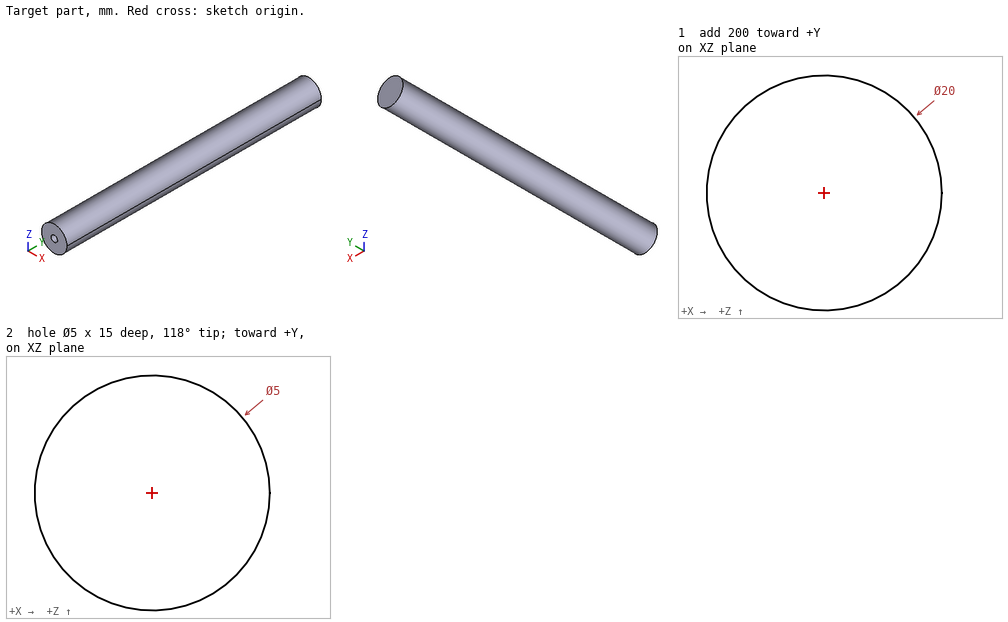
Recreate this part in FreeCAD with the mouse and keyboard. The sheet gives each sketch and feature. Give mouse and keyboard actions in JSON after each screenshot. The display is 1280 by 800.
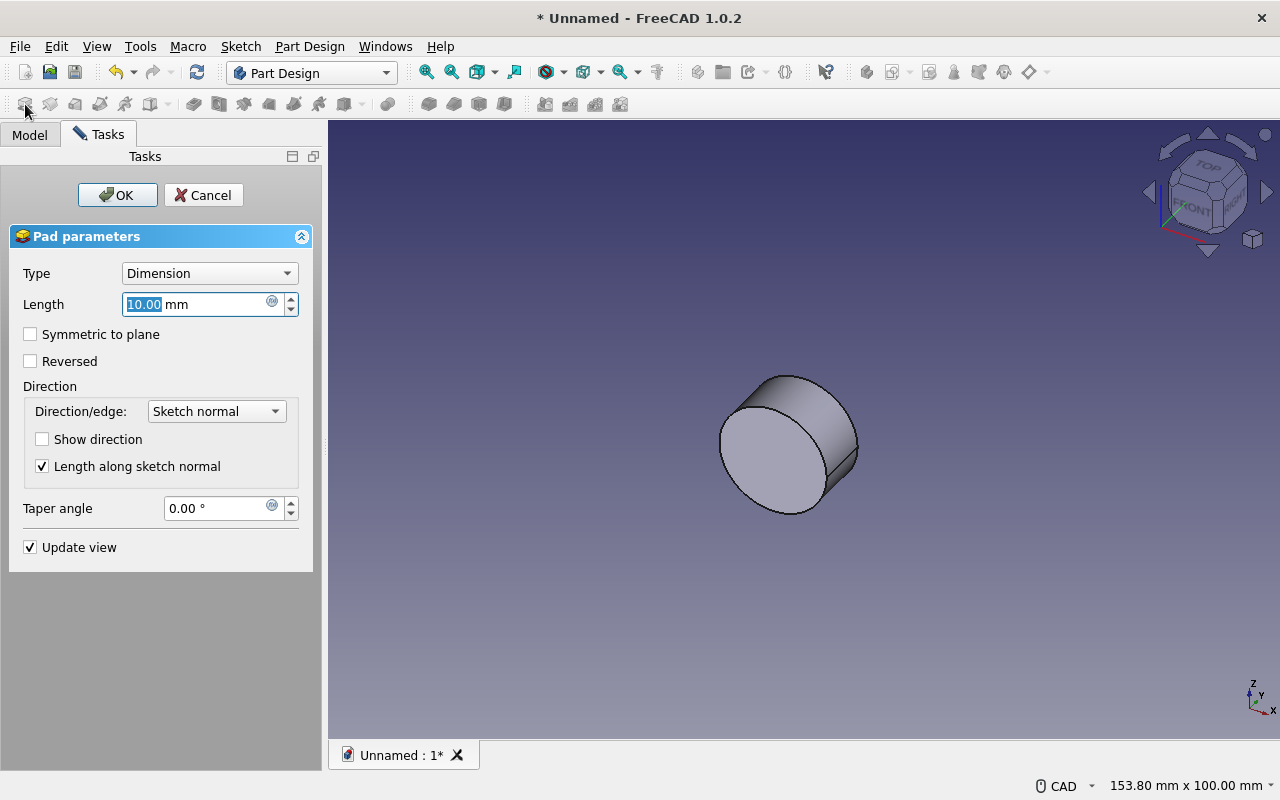
{"action": "type", "text": "200"}
{"action": "key", "text": "Tab"}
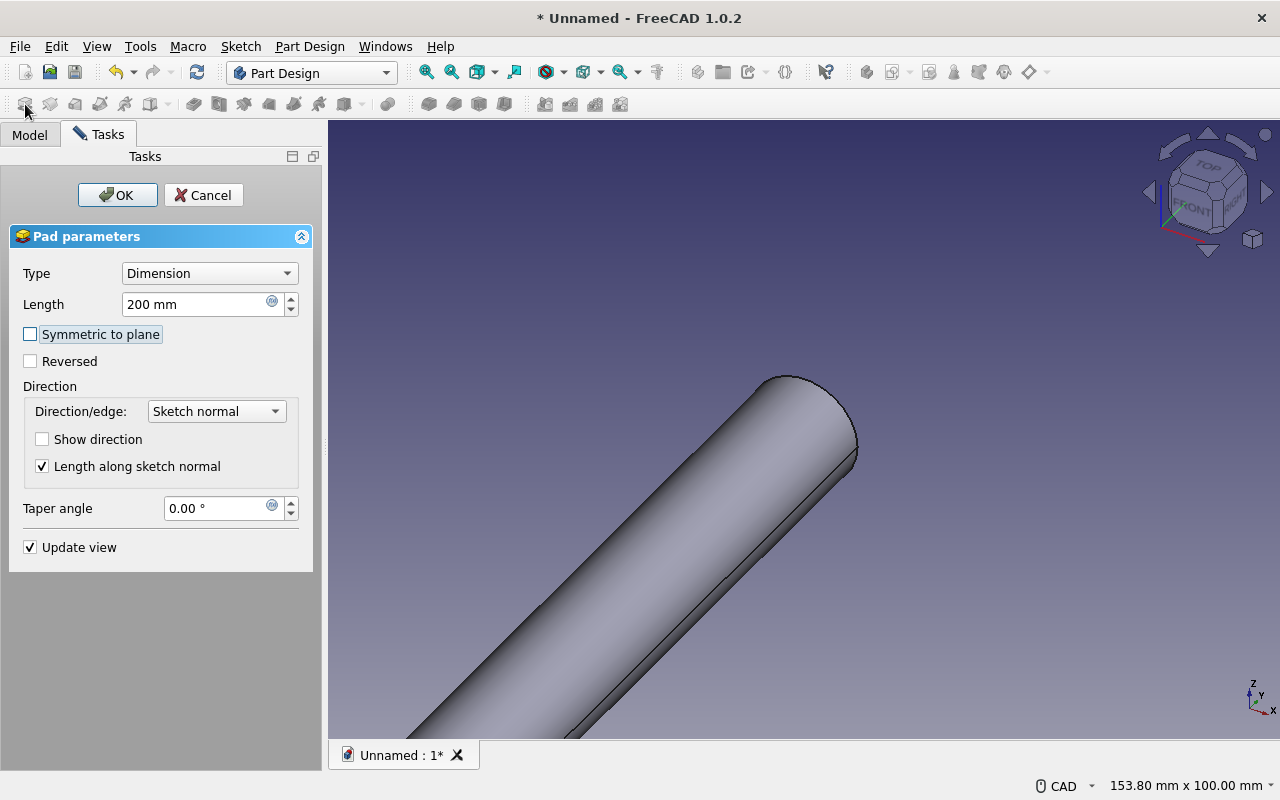
{"action": "left_click", "coordinate": [31, 361]}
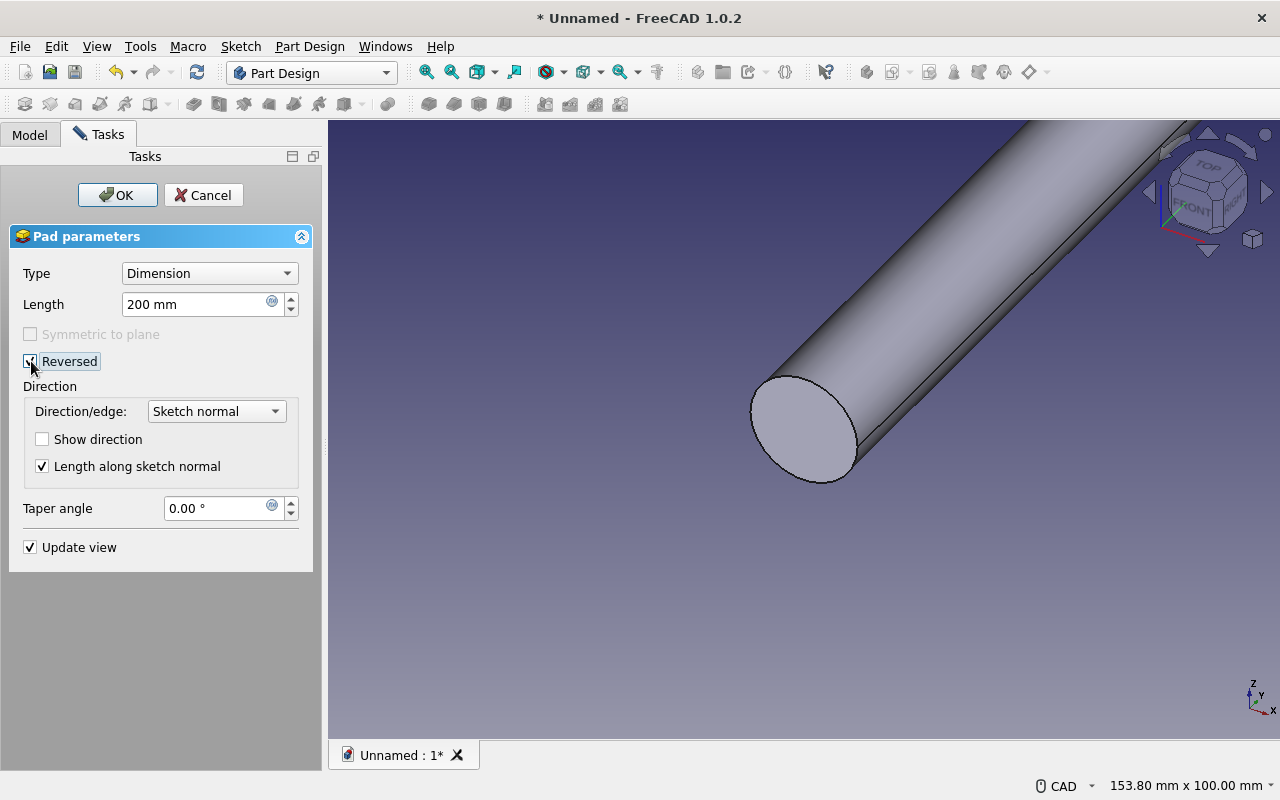
{"action": "left_click", "coordinate": [118, 195]}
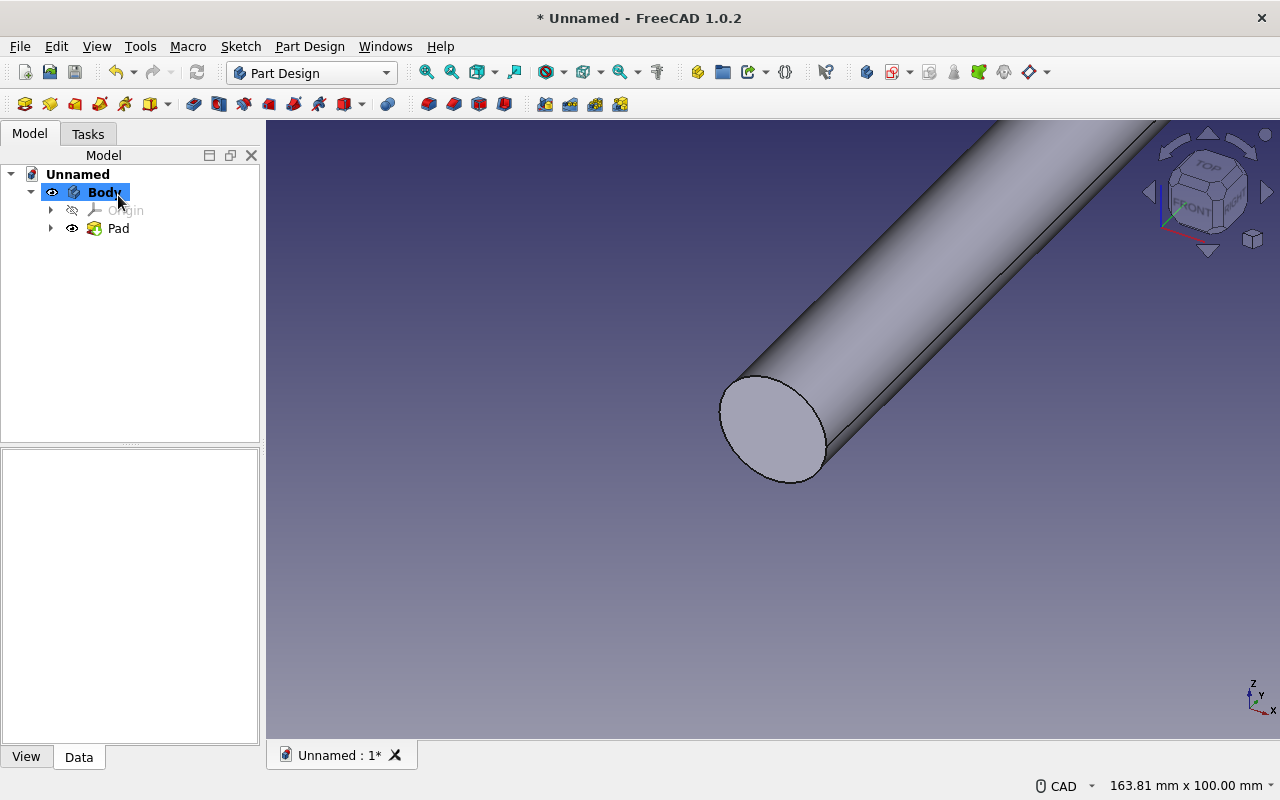
{"action": "left_click", "coordinate": [427, 72]}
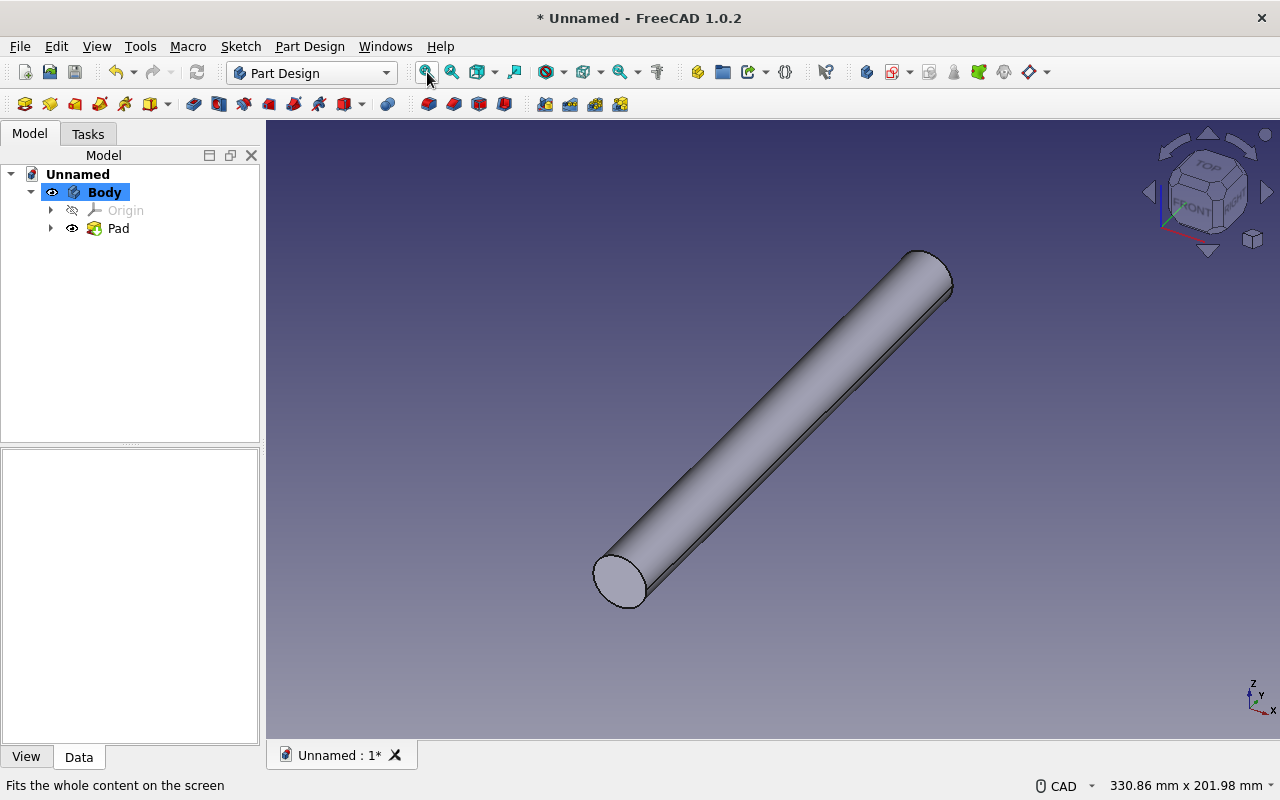
{"action": "left_click", "coordinate": [892, 72]}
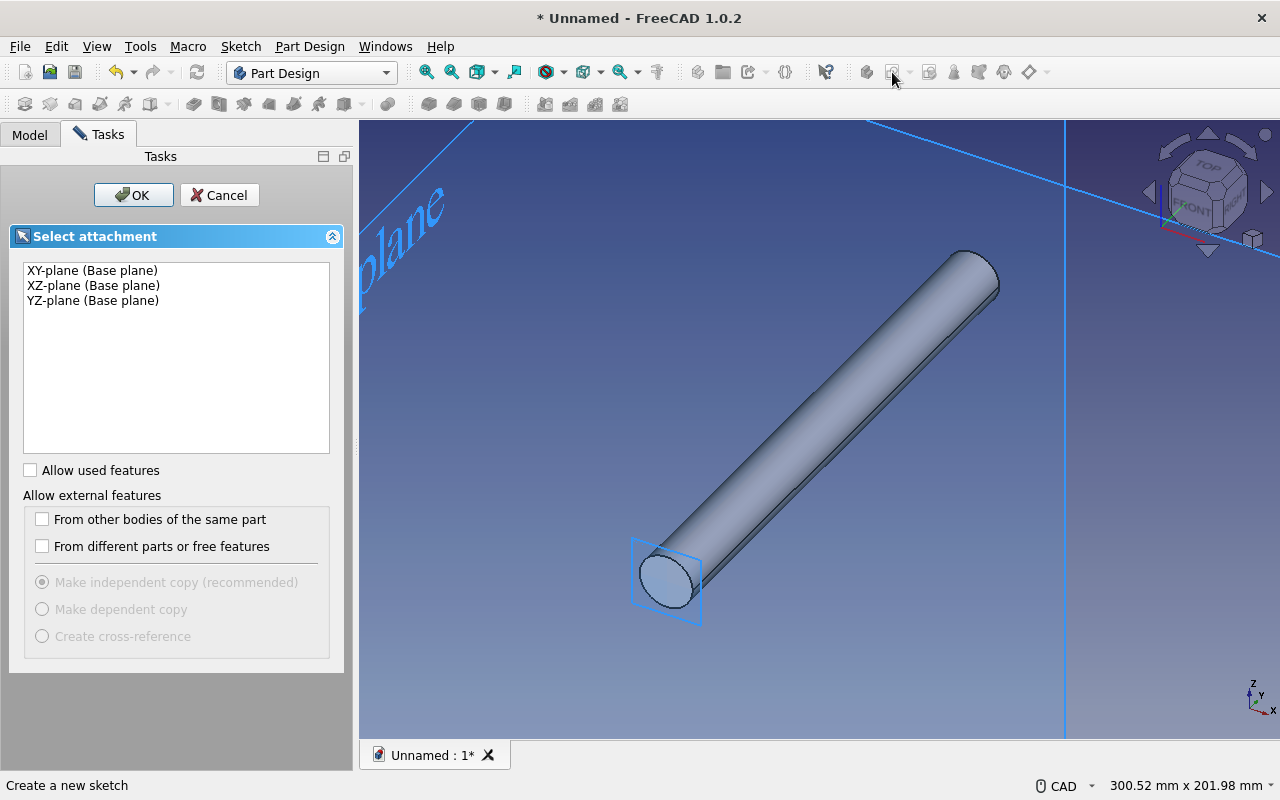
{"action": "left_click", "coordinate": [84, 286]}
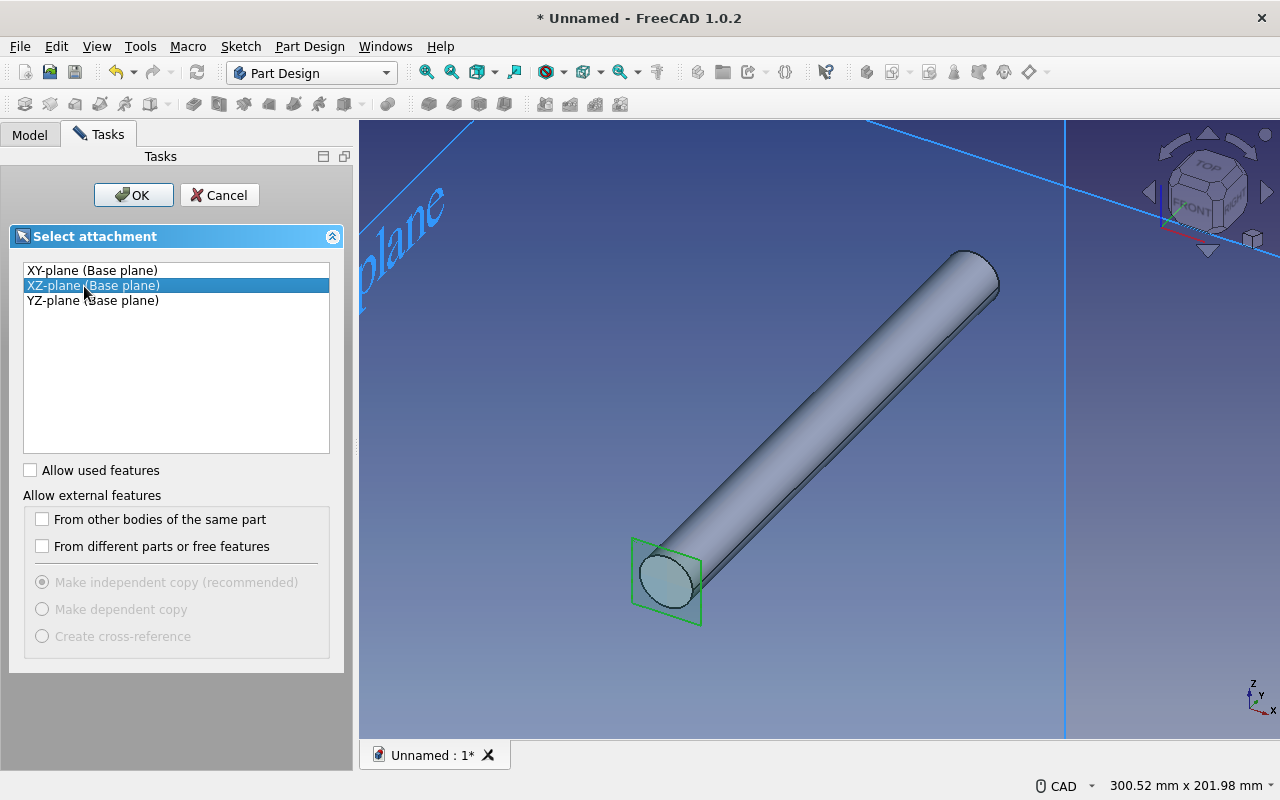
{"action": "left_click", "coordinate": [134, 195]}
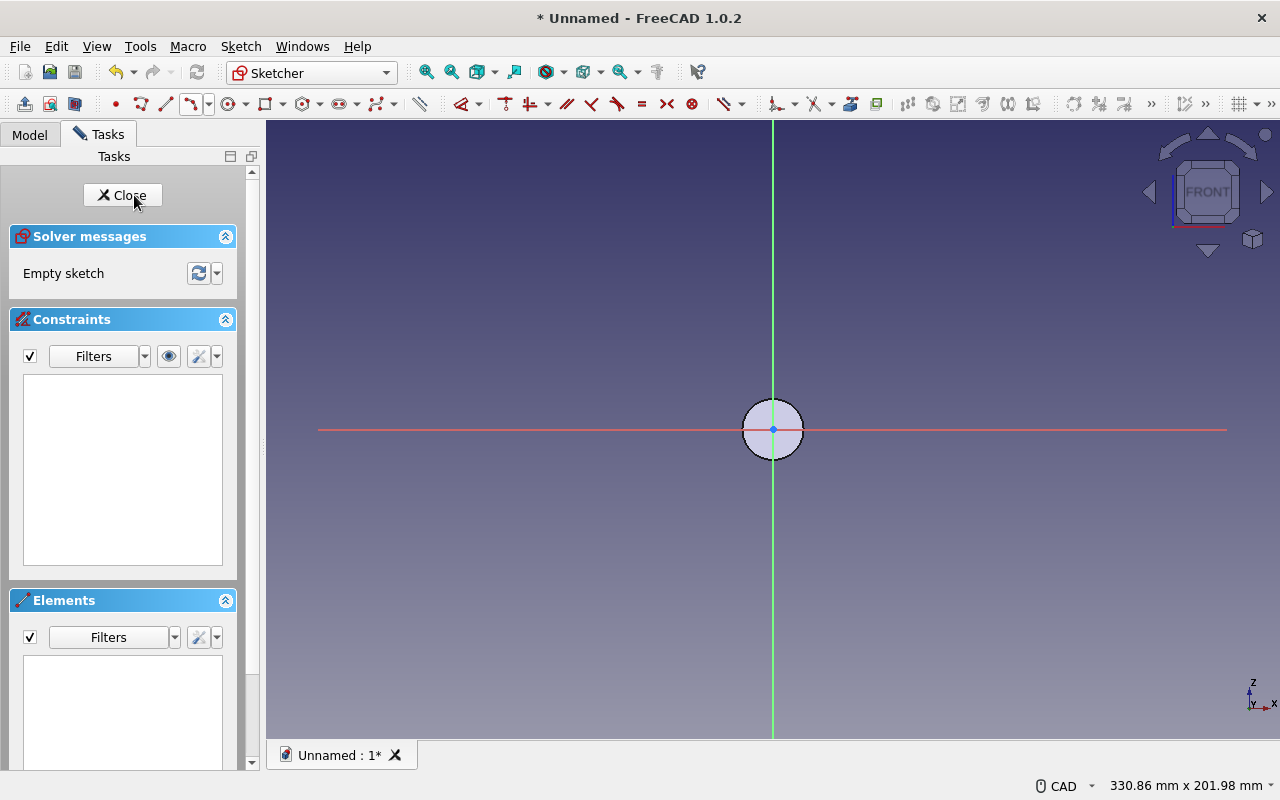
{"action": "scroll", "coordinate": [777, 430], "scroll_direction": "up", "scroll_amount": 15}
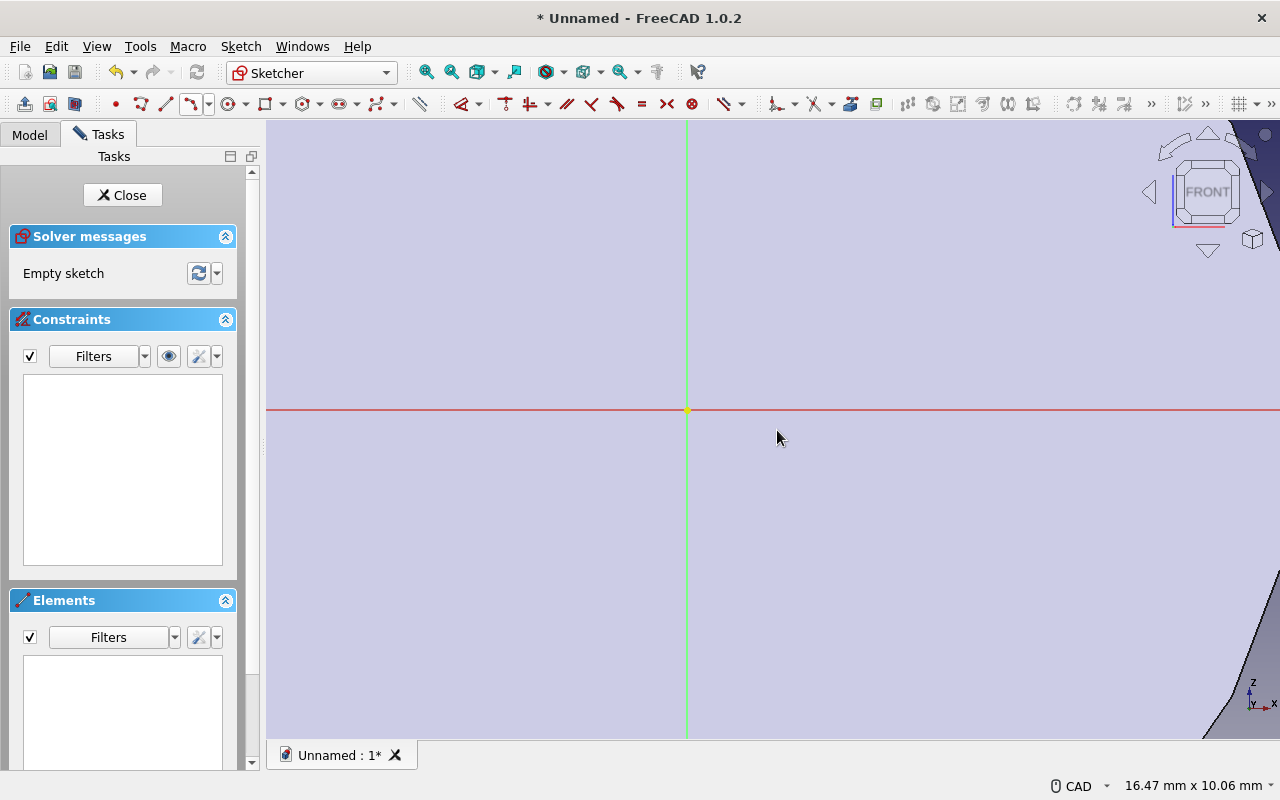
{"action": "left_click", "coordinate": [228, 104]}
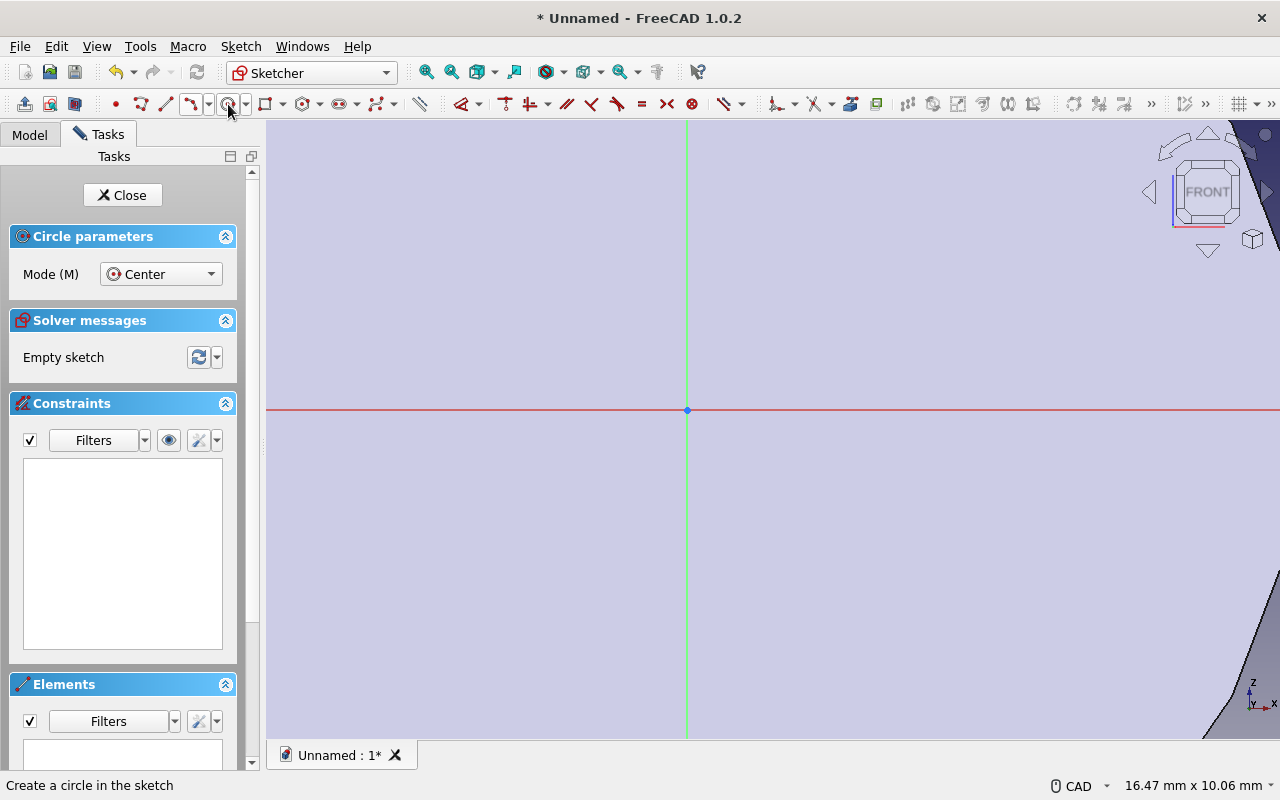
{"action": "left_click", "coordinate": [687, 410]}
{"action": "mouse_move", "coordinate": [796, 302]}